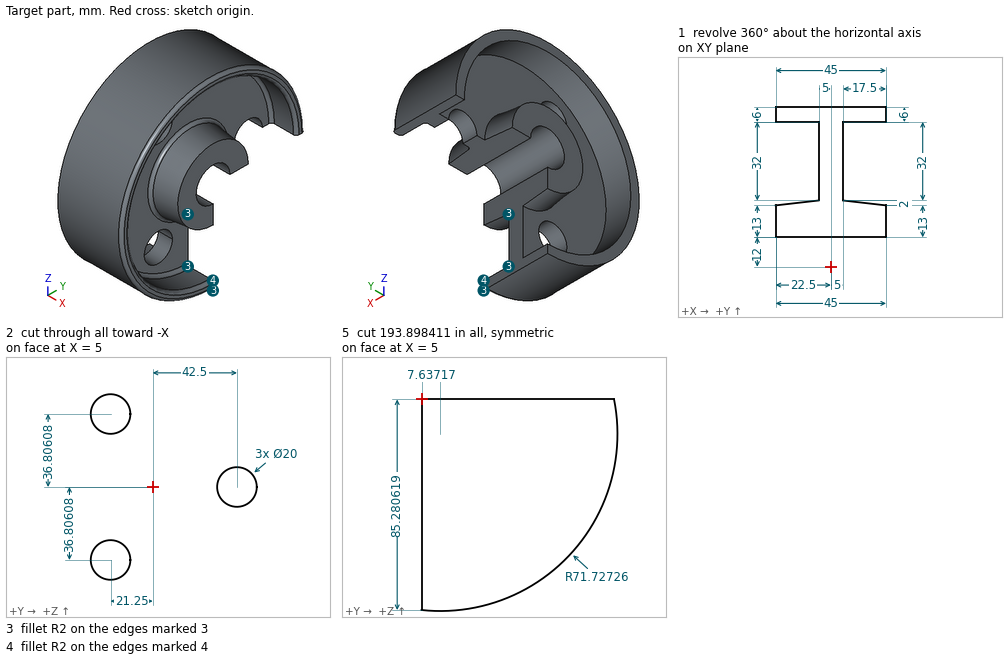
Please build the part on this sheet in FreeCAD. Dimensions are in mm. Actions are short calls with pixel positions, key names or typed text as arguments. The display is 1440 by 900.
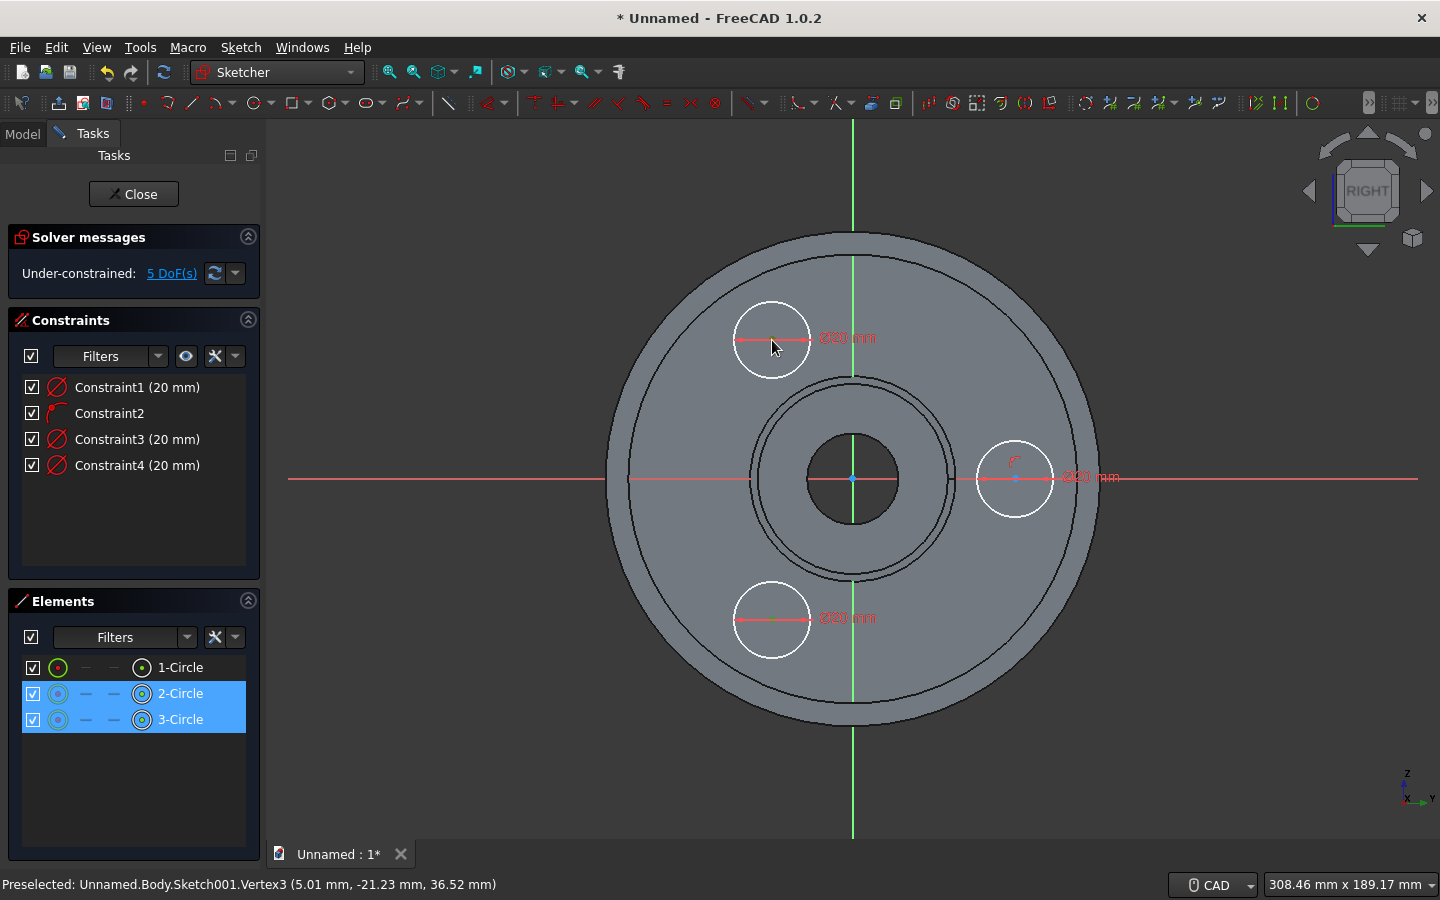
click(576, 104)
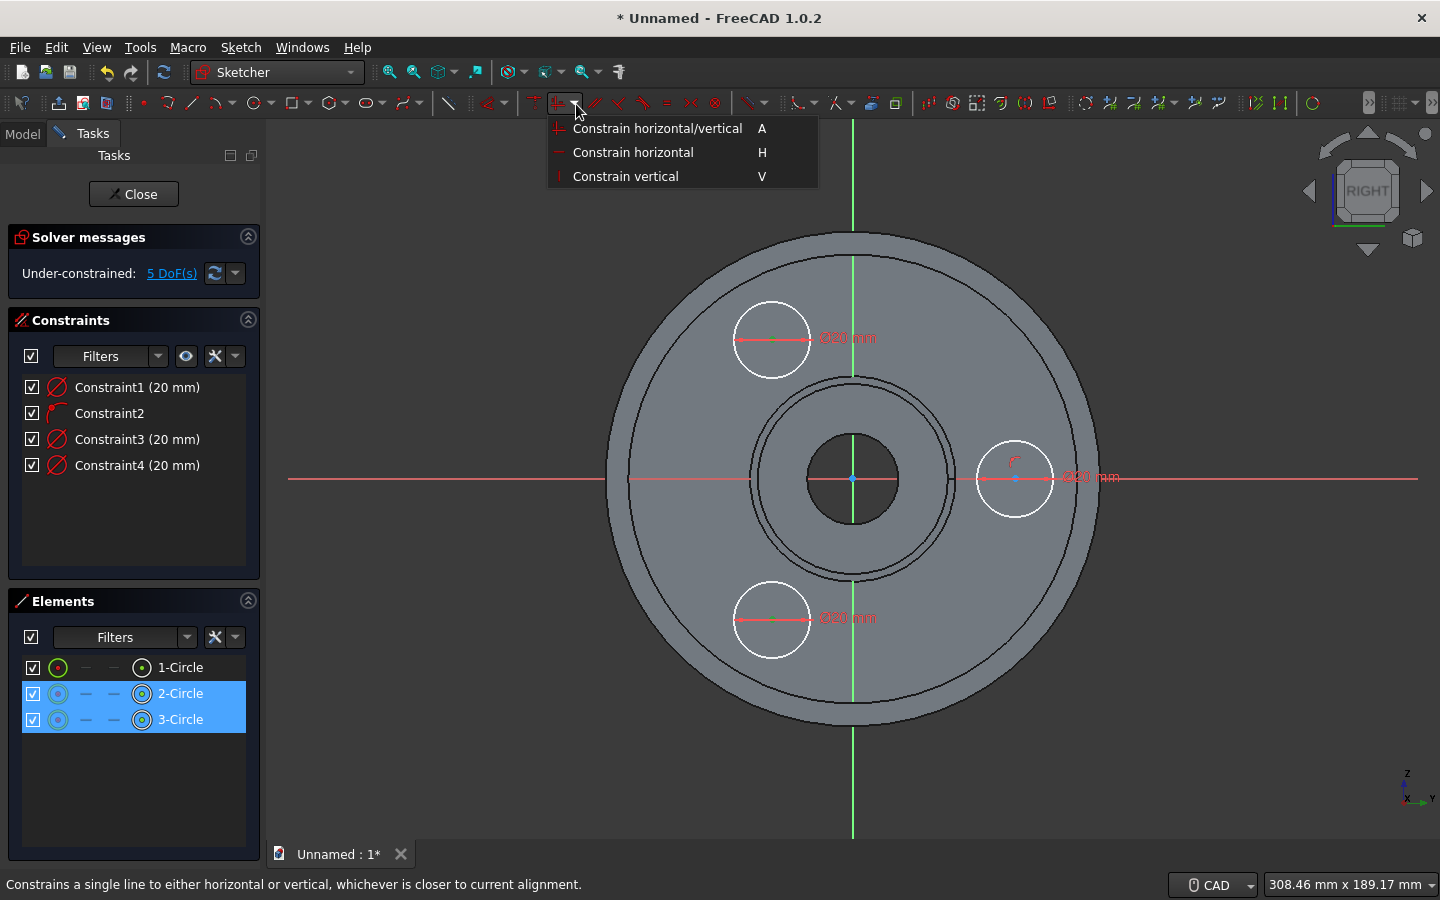
click(683, 176)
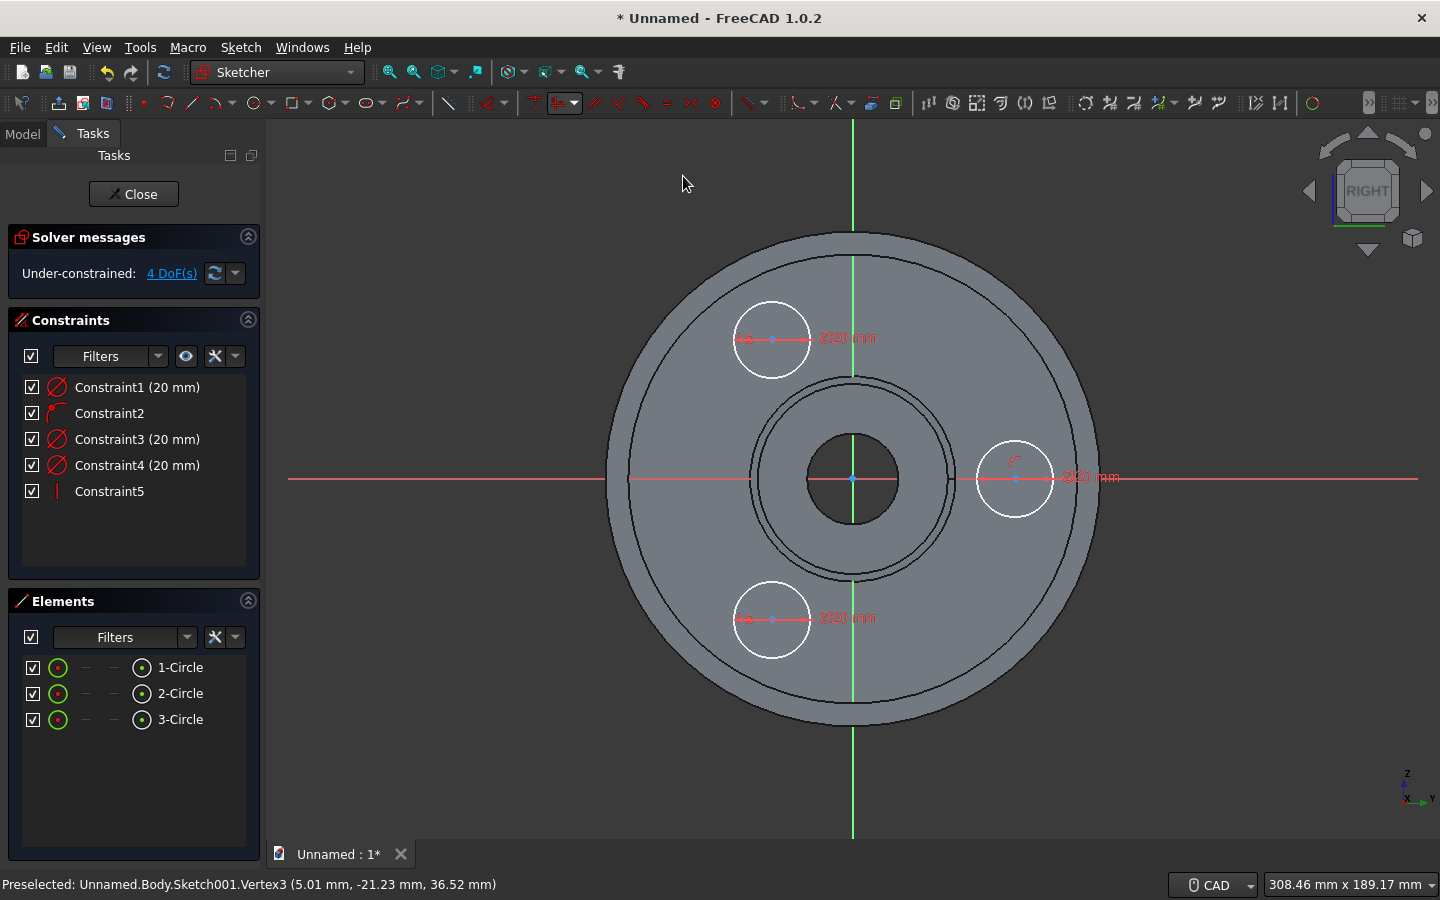
click(488, 104)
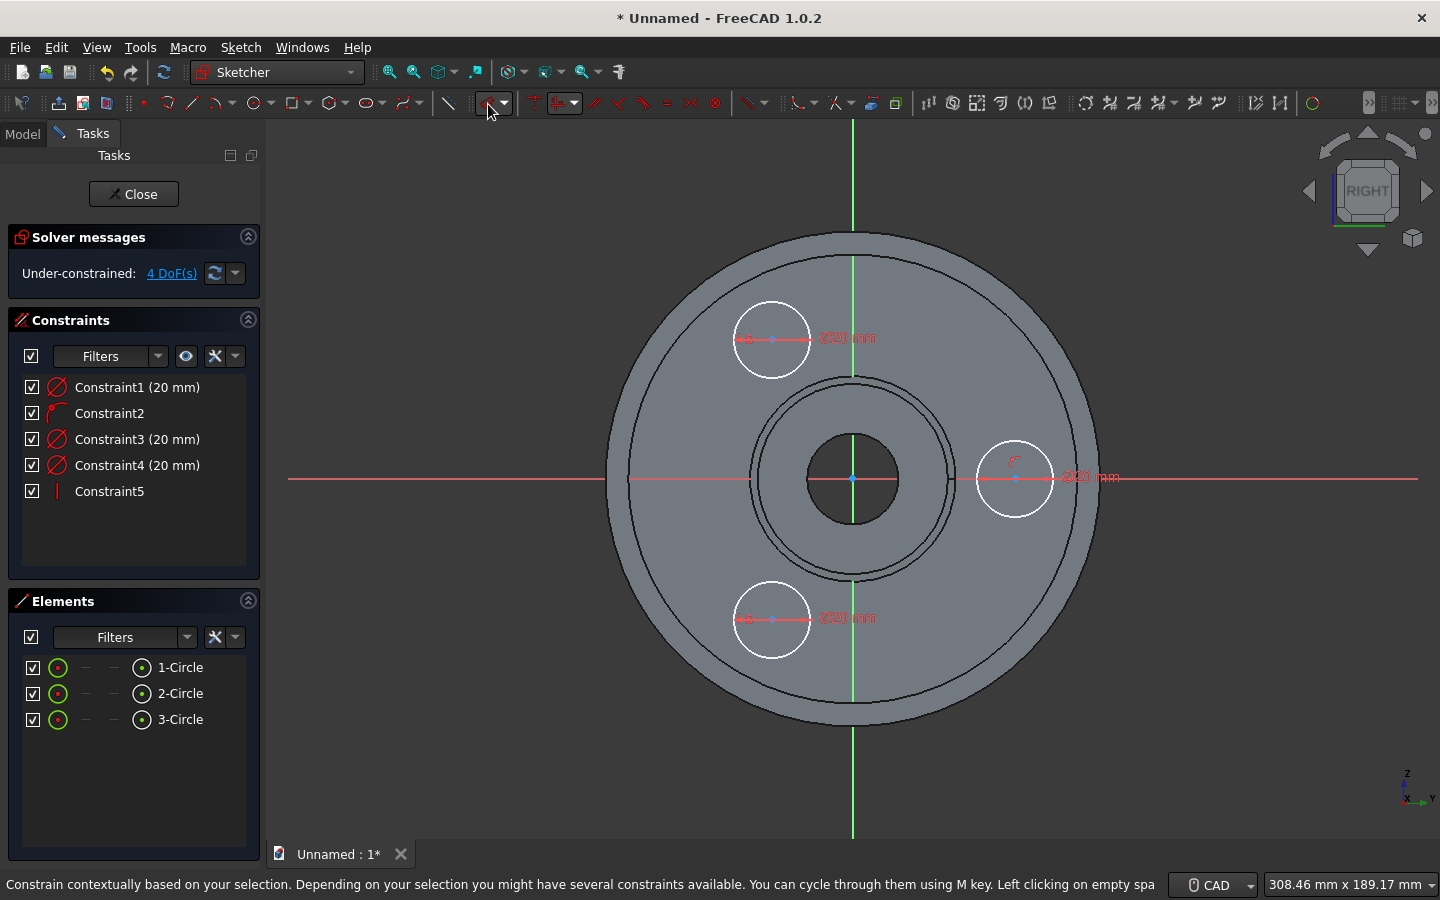
click(1015, 479)
click(934, 513)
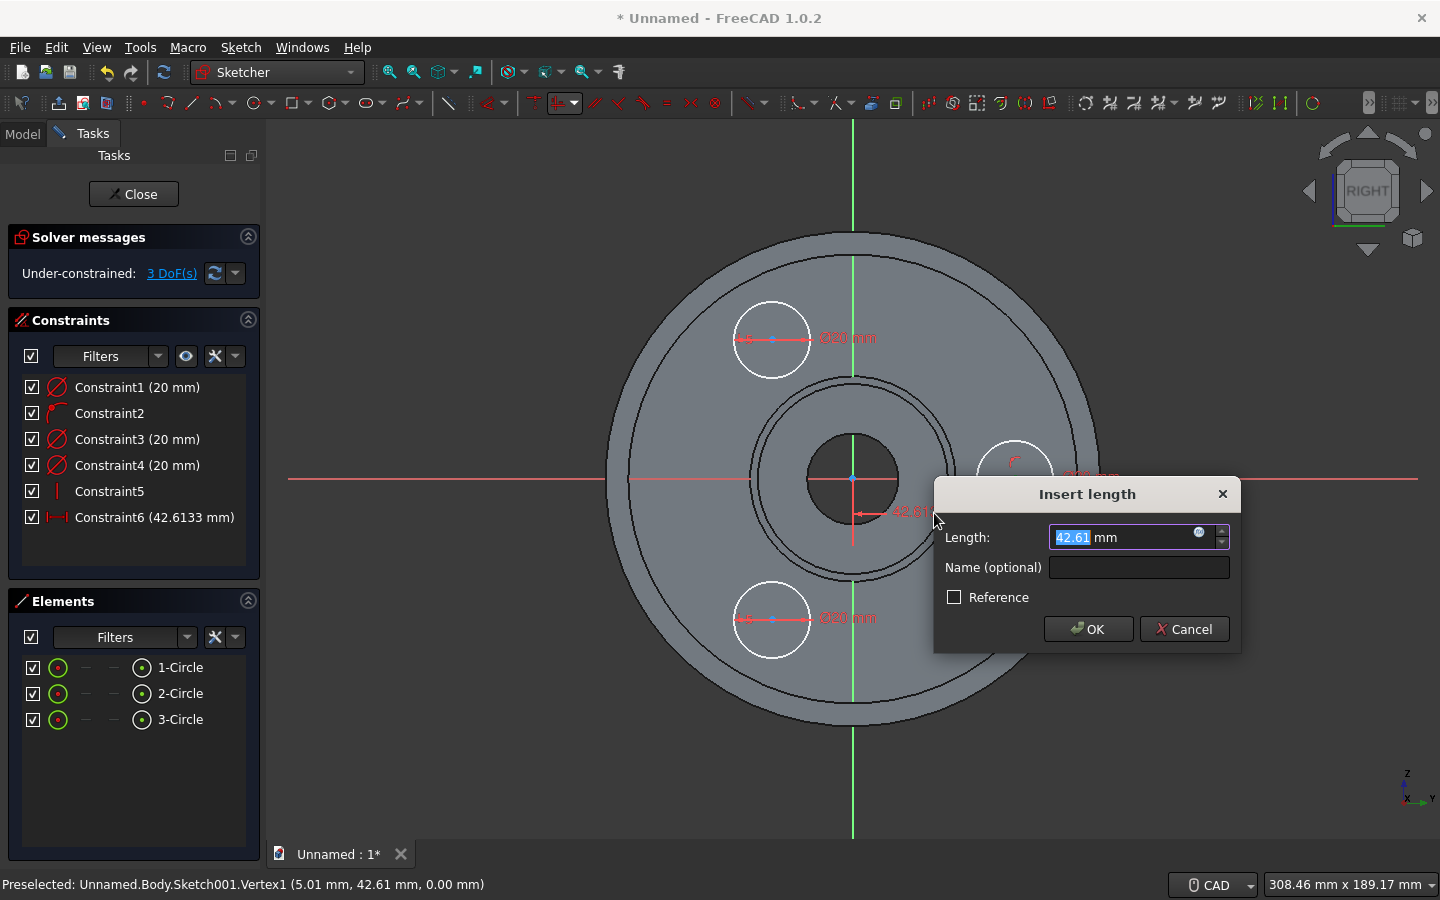
text(42.5)
key(Return)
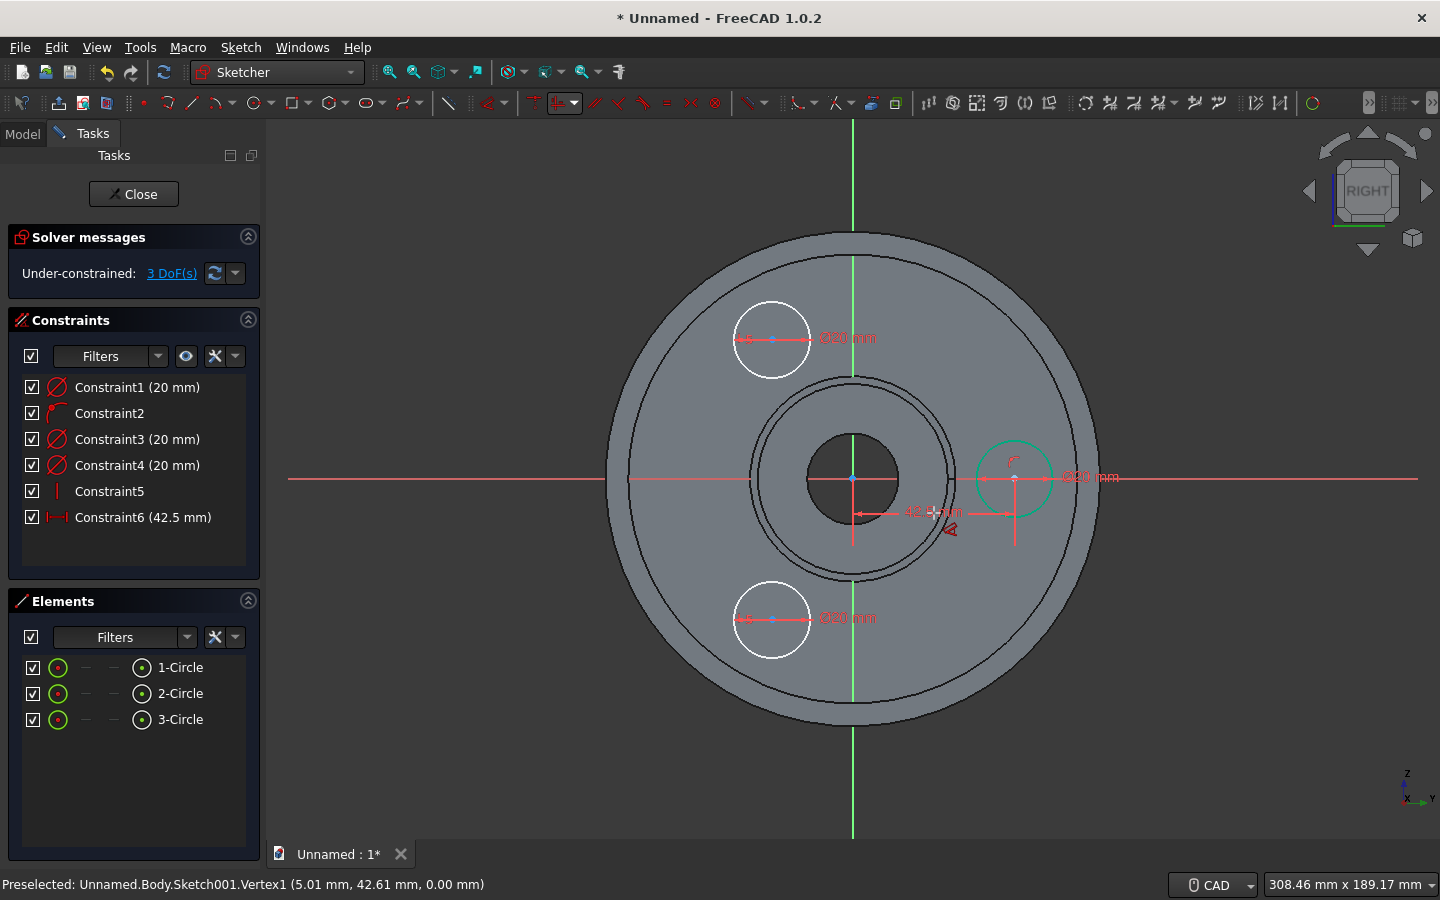
click(772, 620)
click(812, 654)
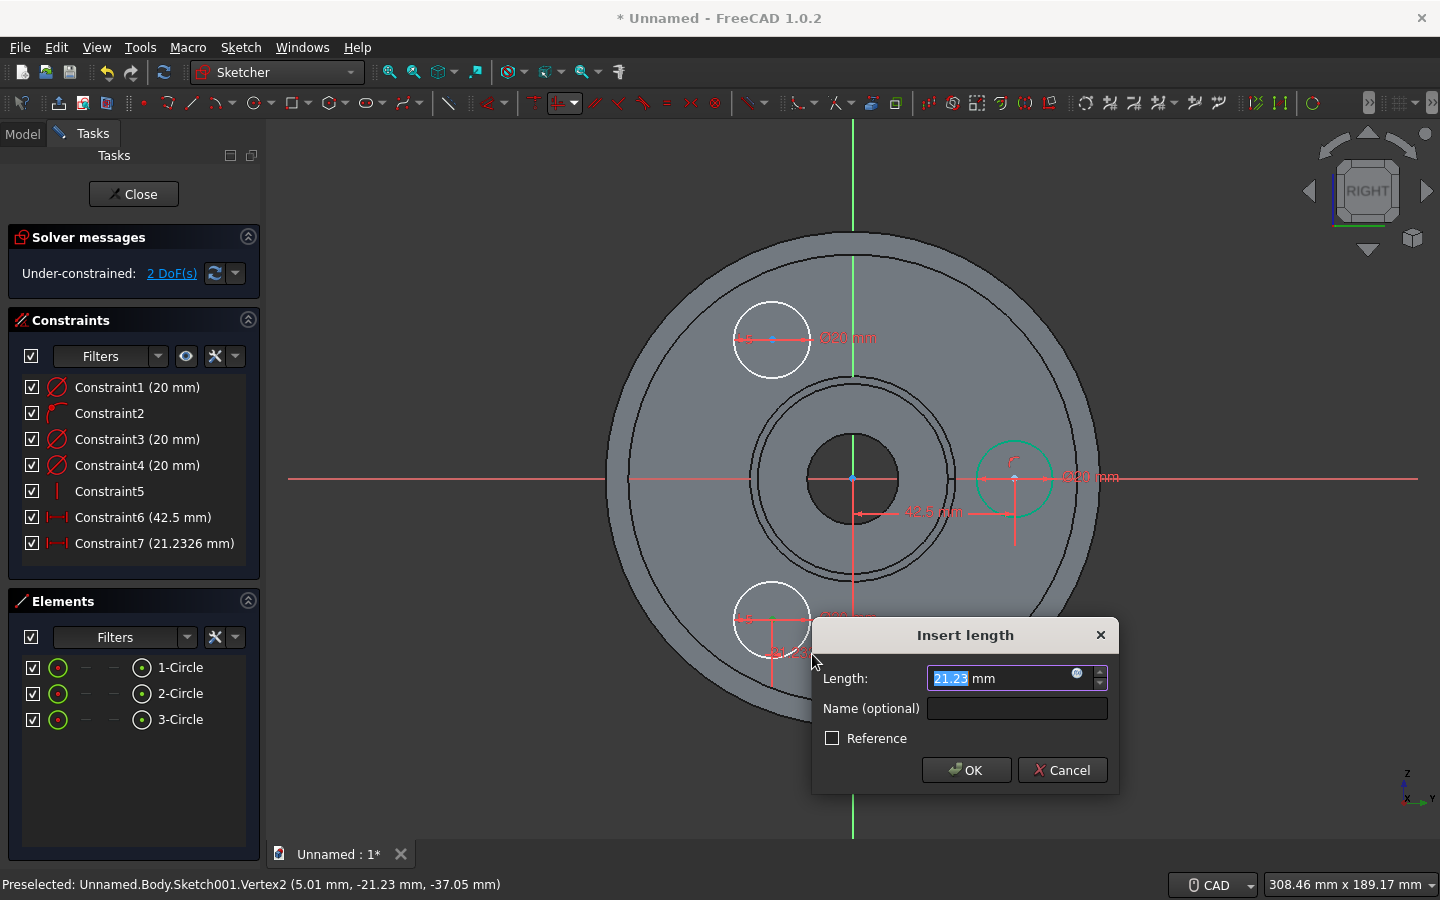
text(21.25)
key(Return)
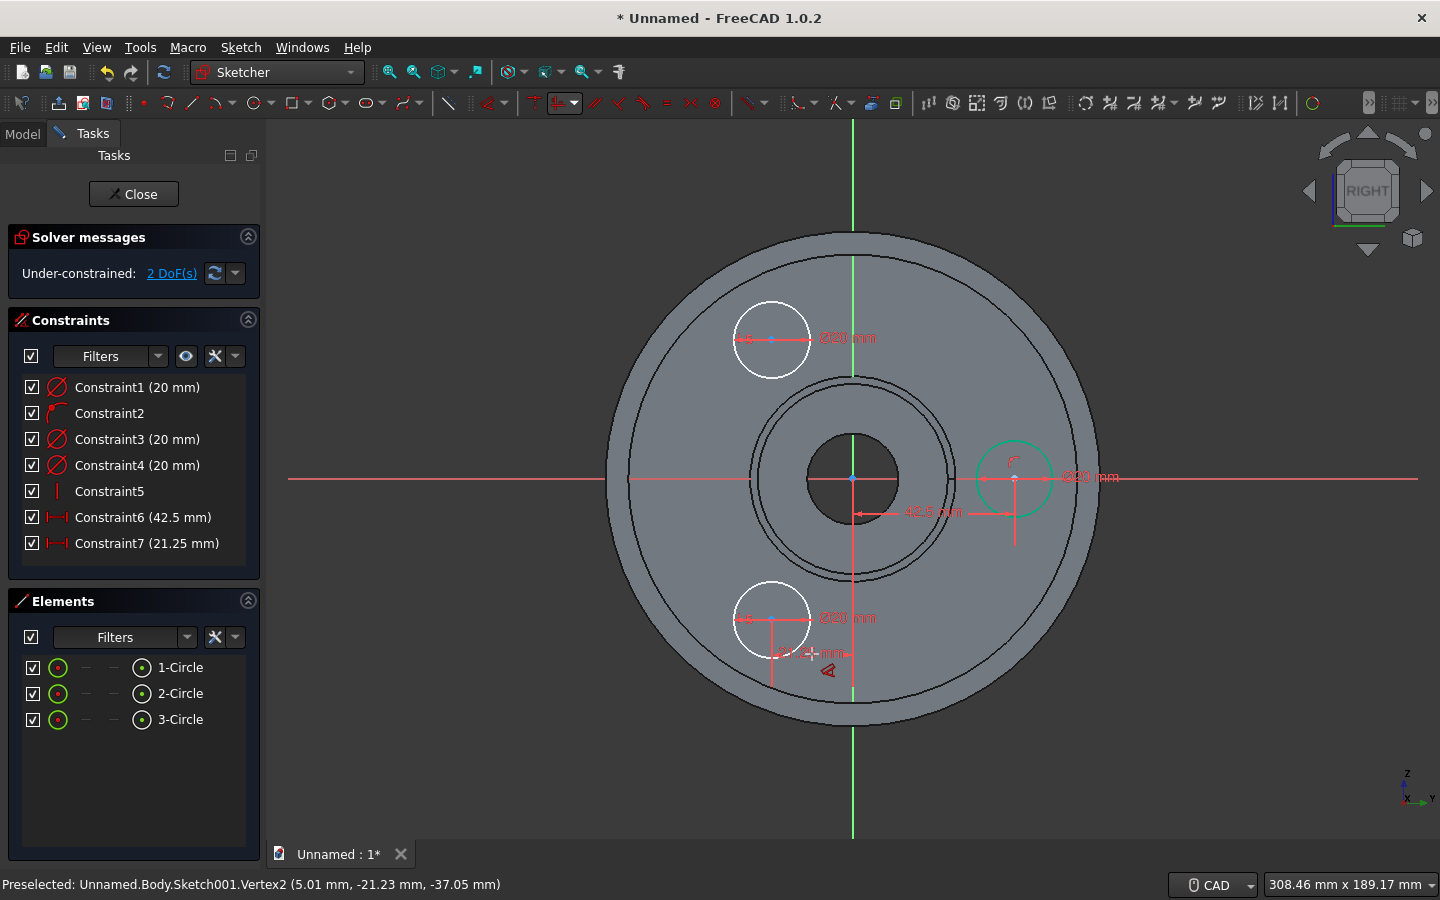
click(772, 620)
click(738, 549)